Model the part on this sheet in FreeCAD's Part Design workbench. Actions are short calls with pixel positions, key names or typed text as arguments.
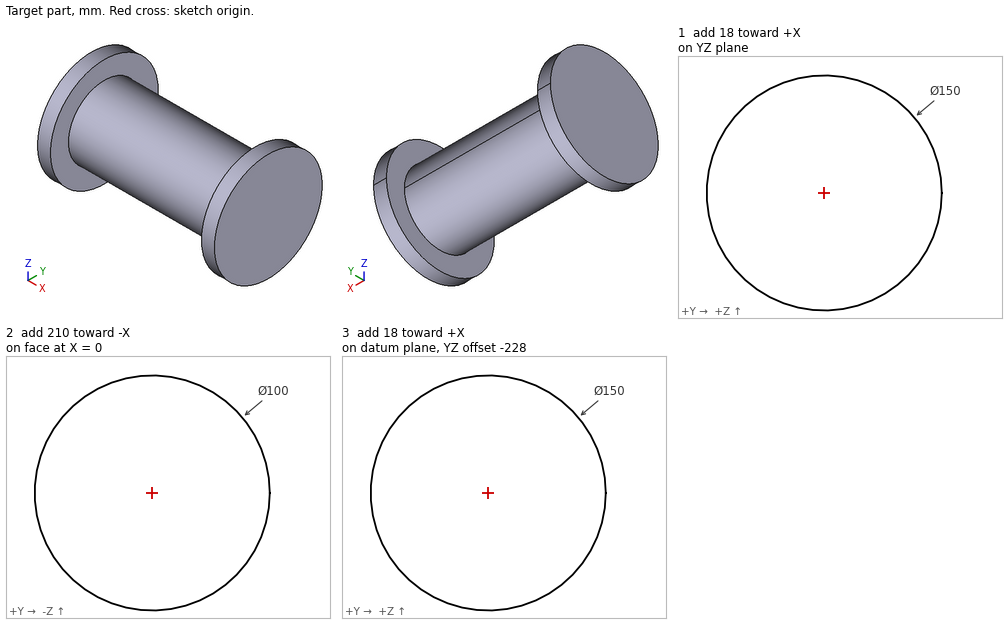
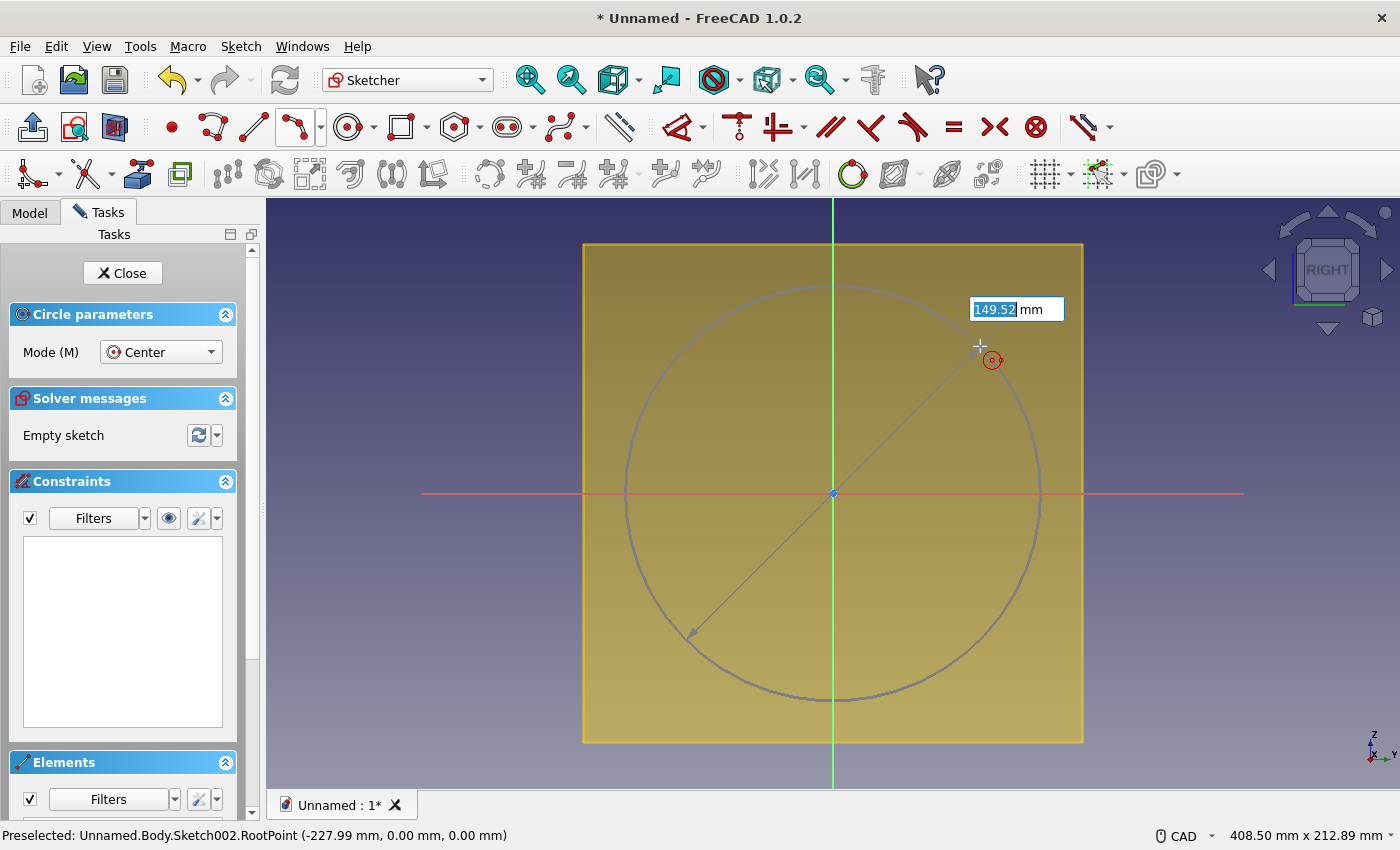
text(150)
key(Return)
key(Escape)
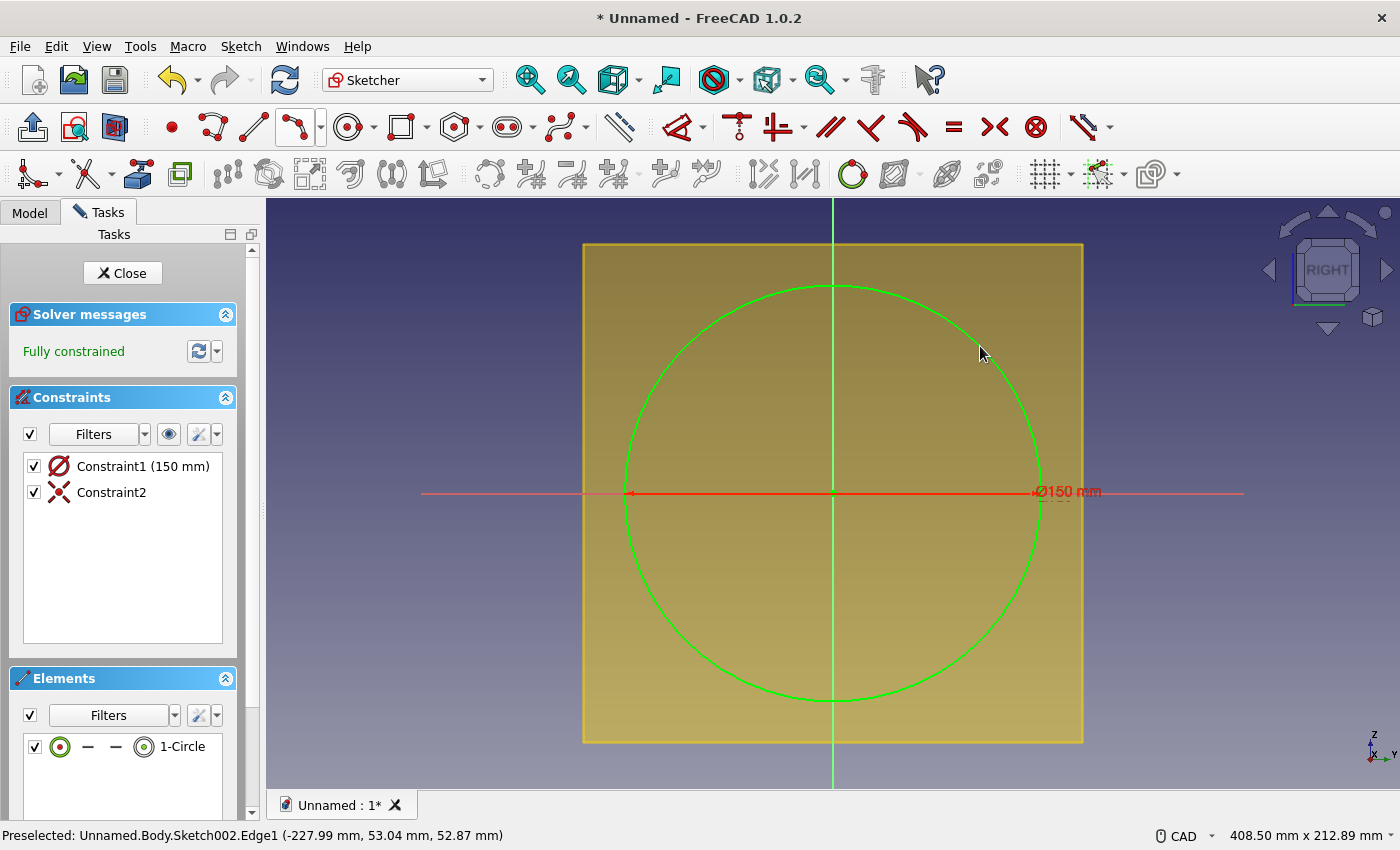
click(123, 273)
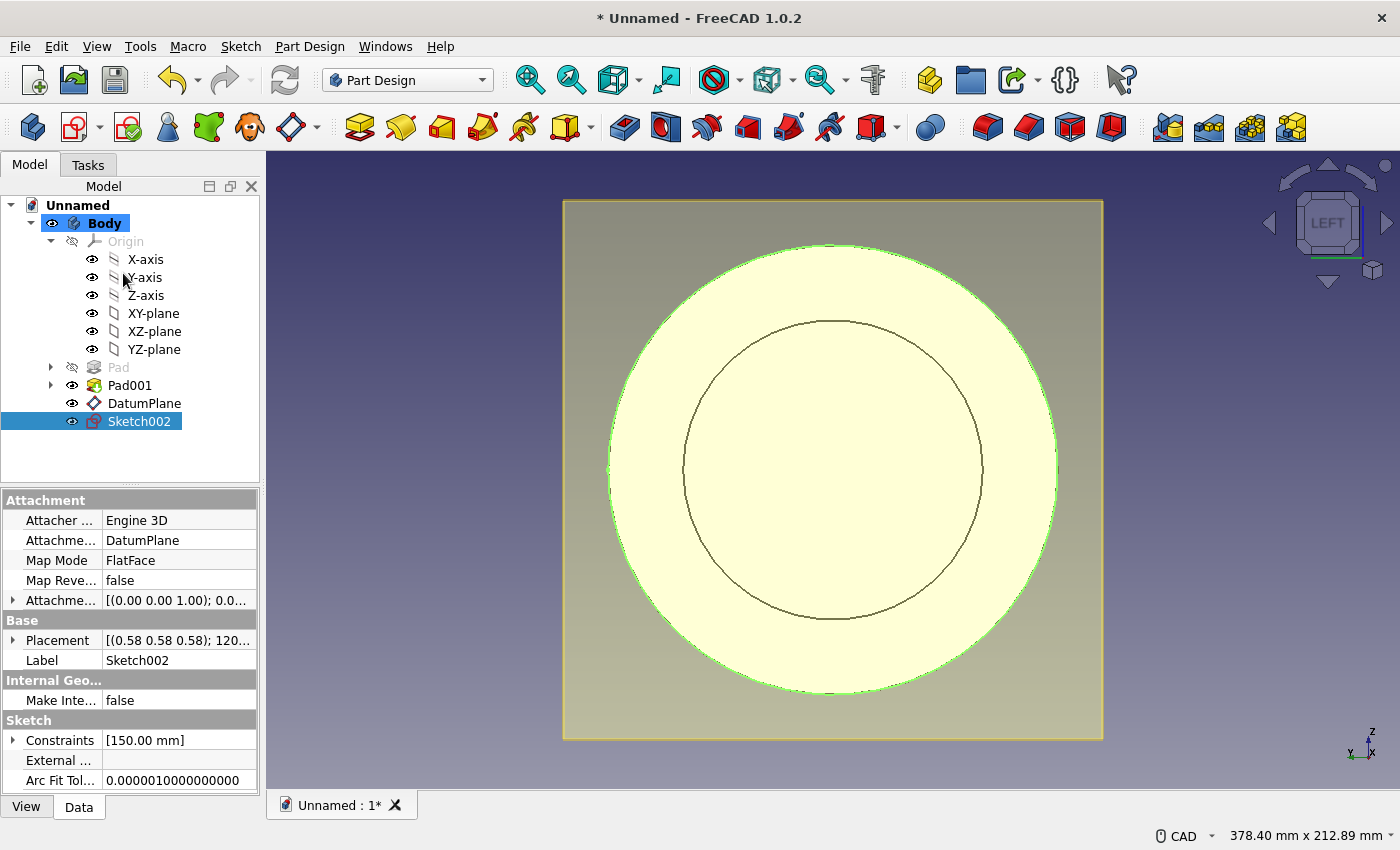
click(360, 128)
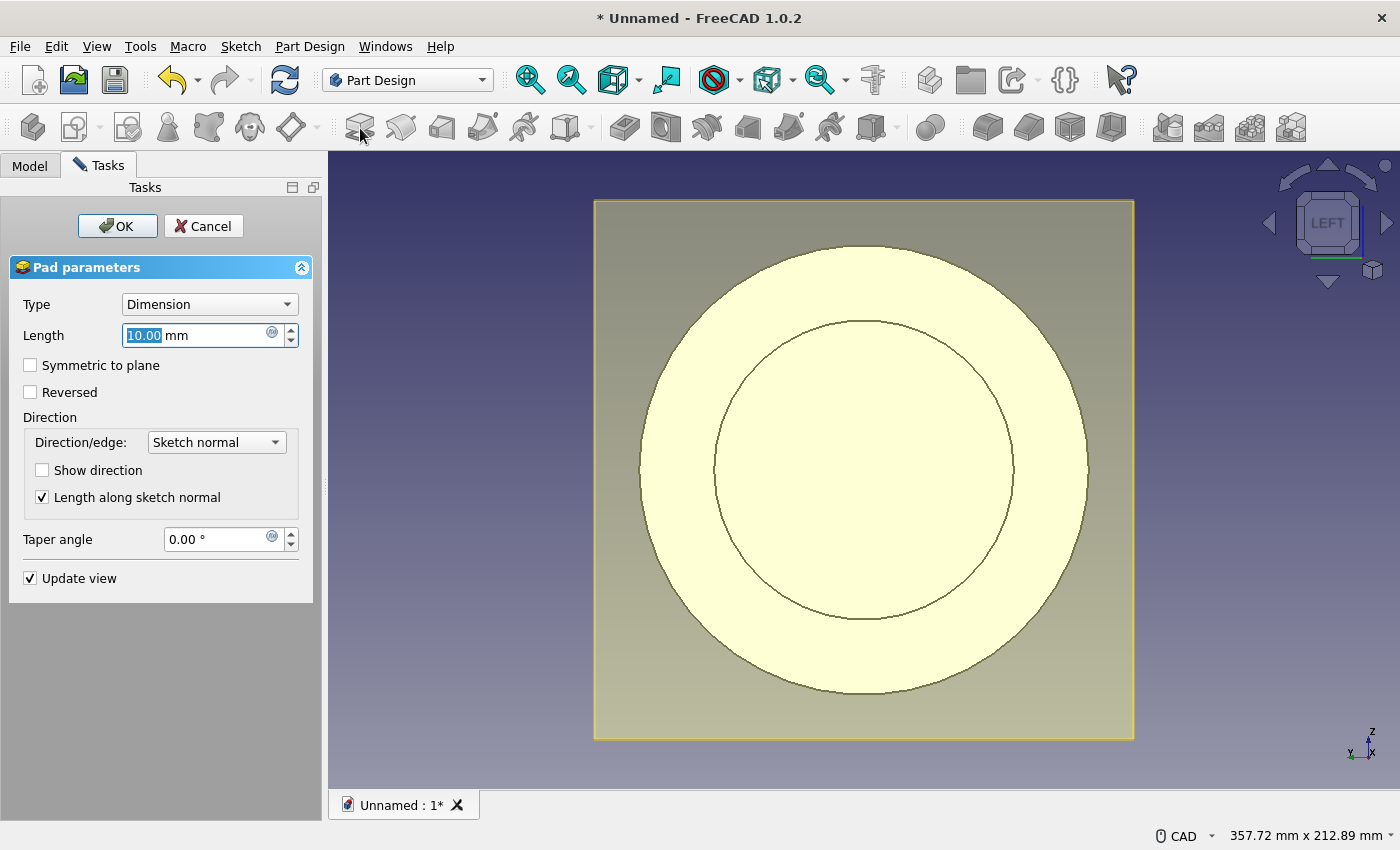
text(18)
key(Tab)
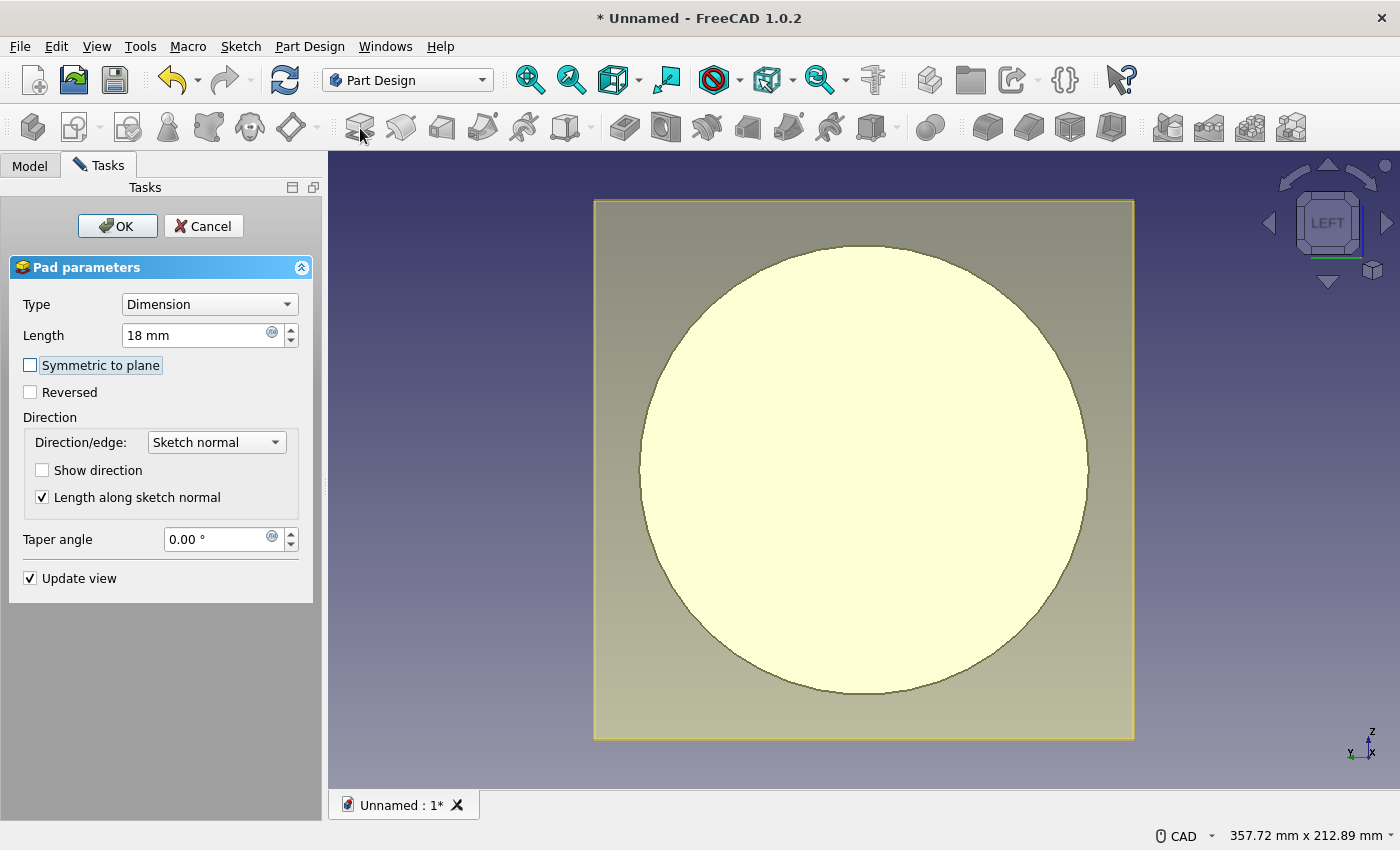
click(118, 226)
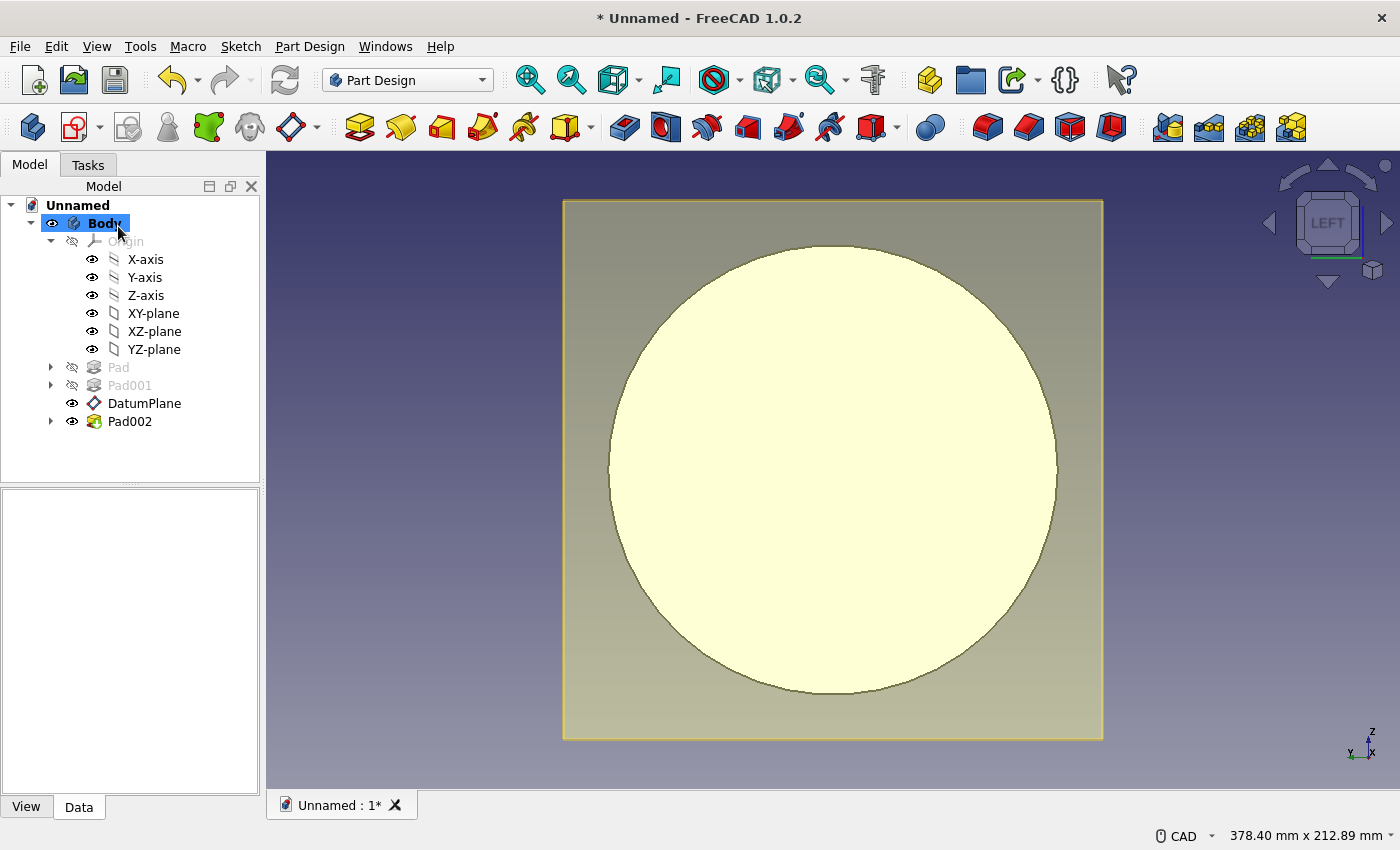
click(117, 403)
key(space)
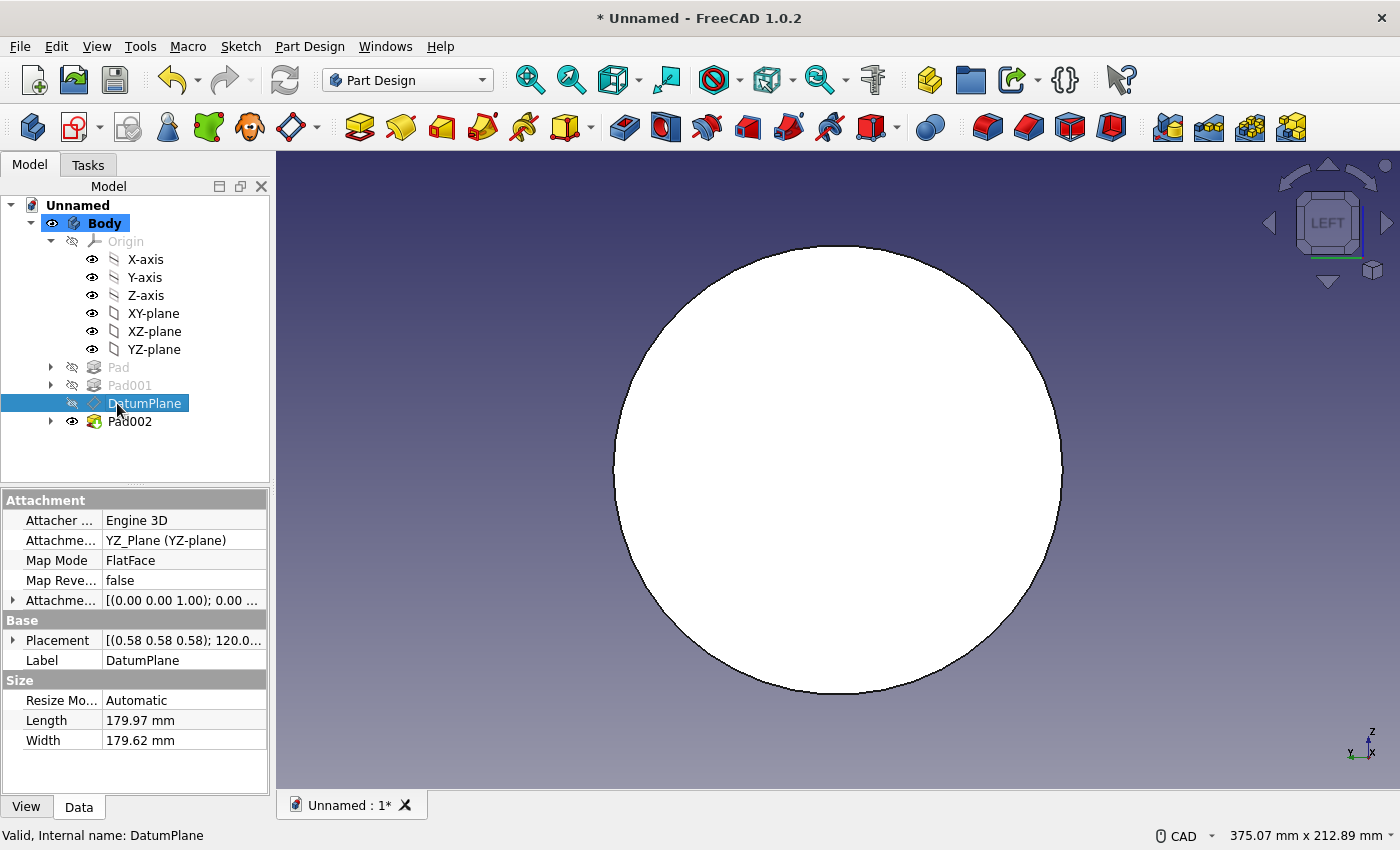
key(0)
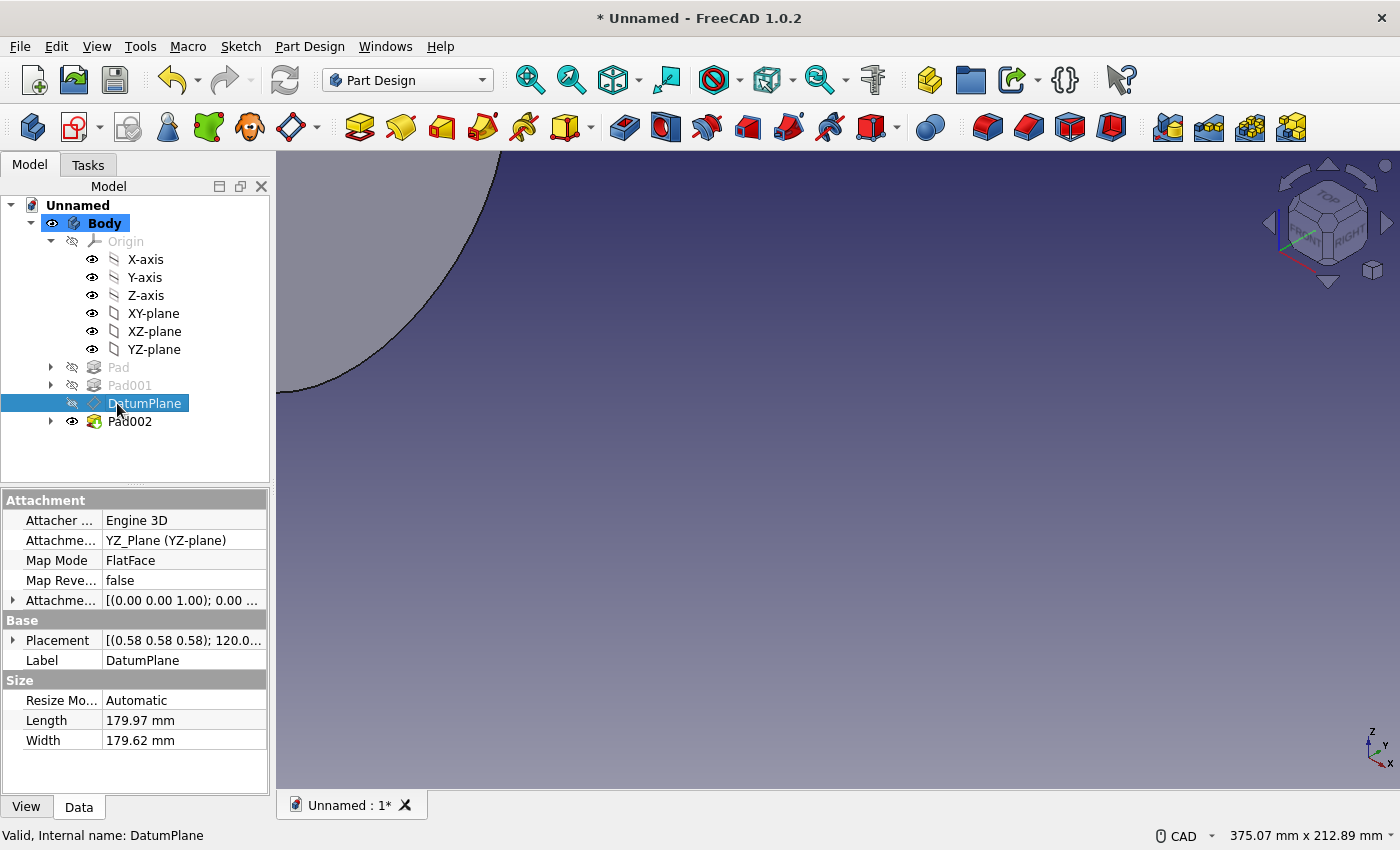
click(531, 80)